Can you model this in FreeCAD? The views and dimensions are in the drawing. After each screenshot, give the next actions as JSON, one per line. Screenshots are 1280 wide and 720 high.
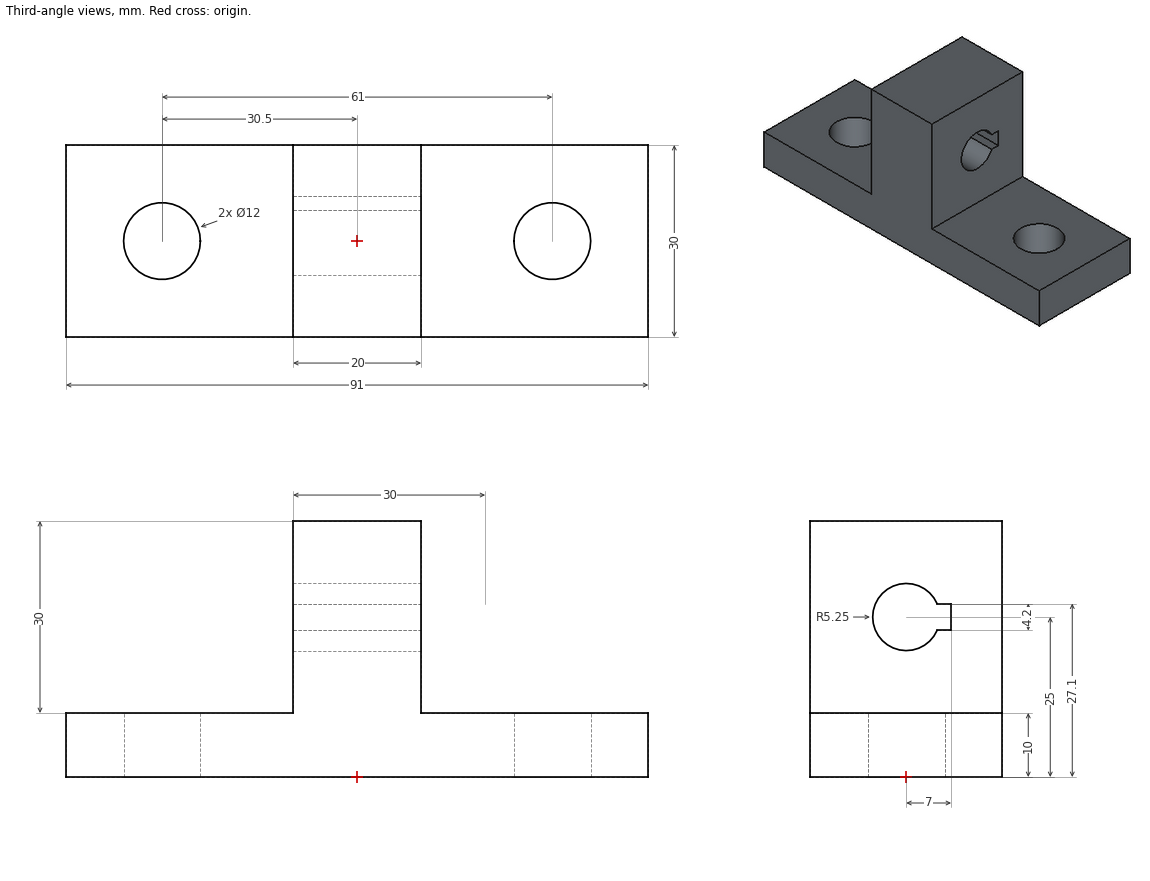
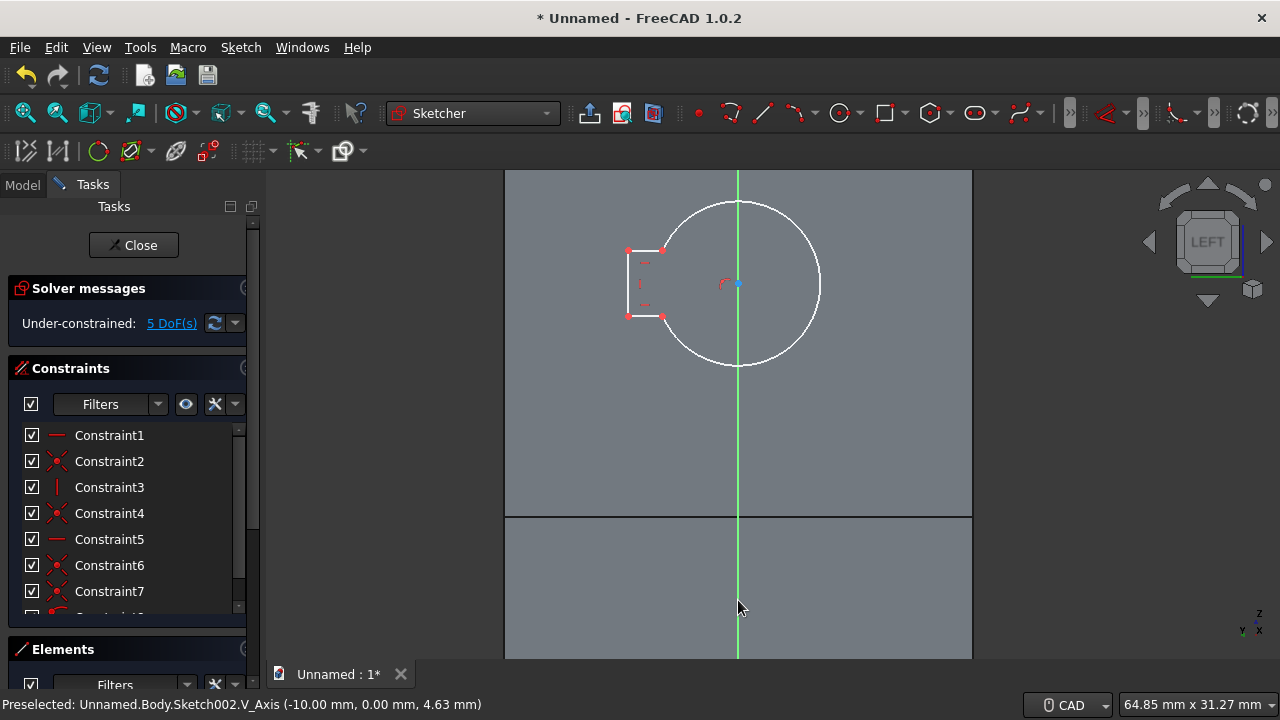
{"action": "left_click", "coordinate": [1106, 114]}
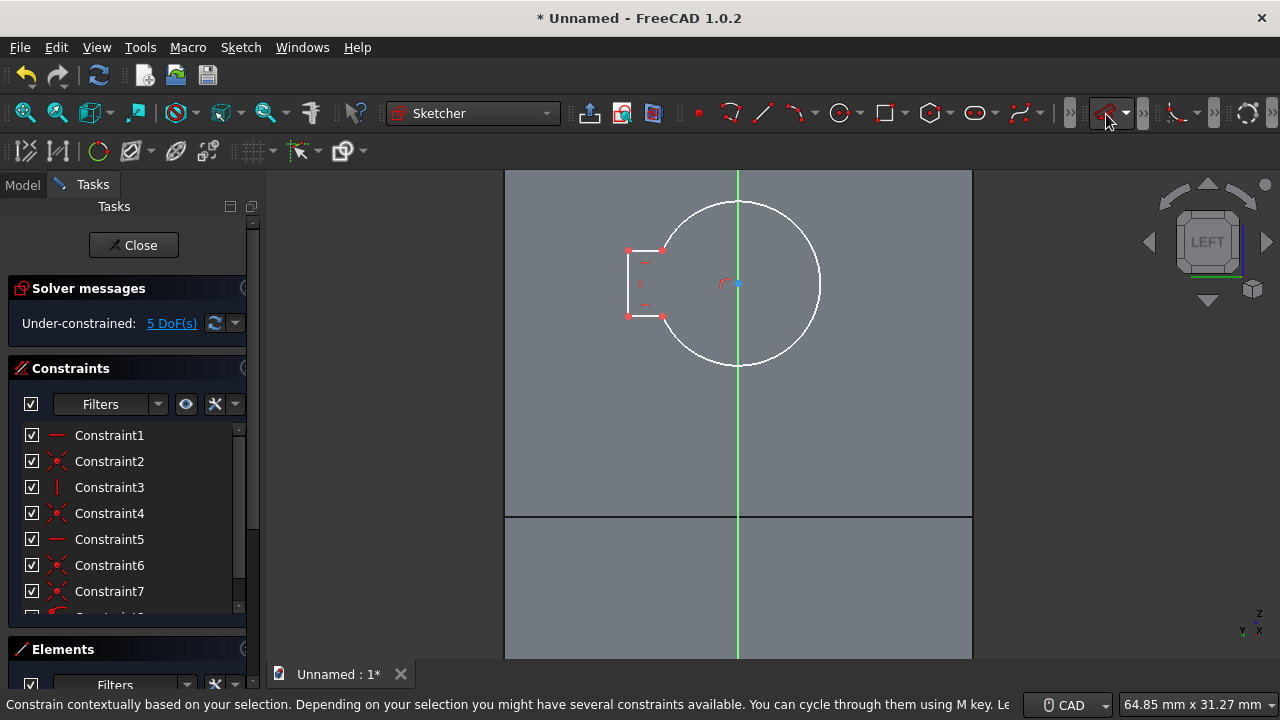
{"action": "left_click", "coordinate": [776, 356]}
{"action": "left_click", "coordinate": [791, 384]}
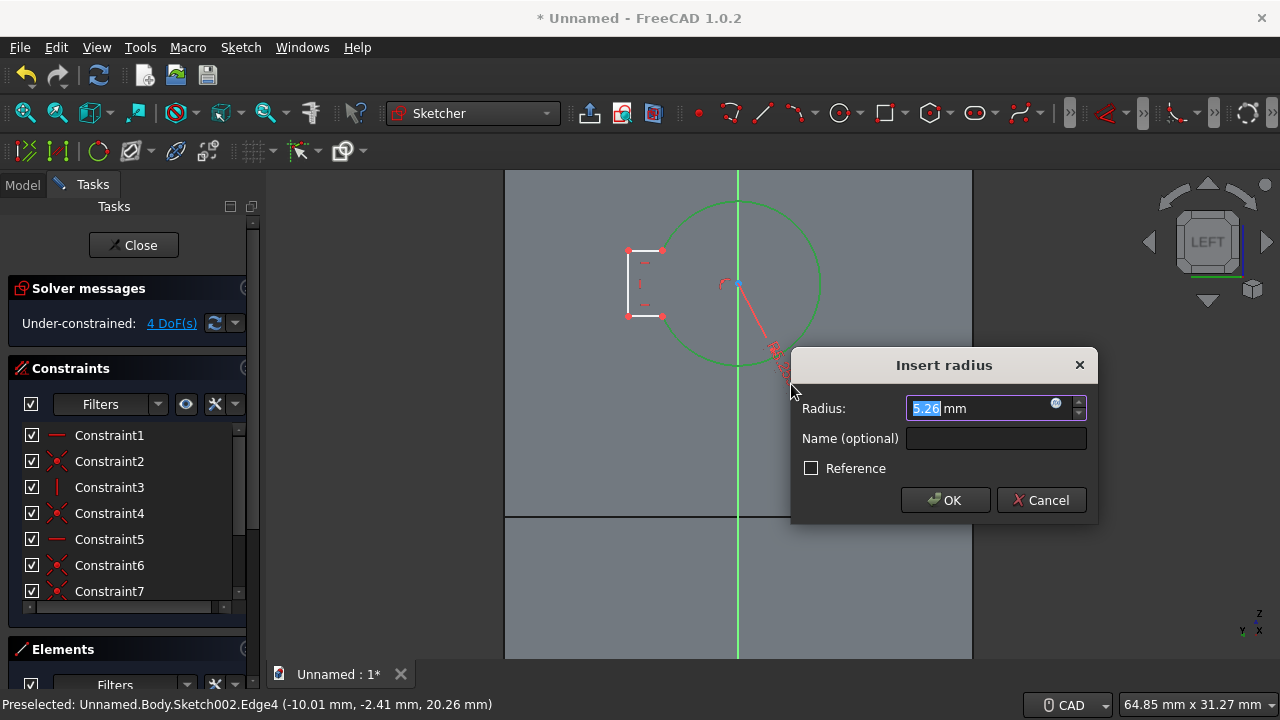
{"action": "type", "text": "5.25"}
{"action": "key", "text": "Return"}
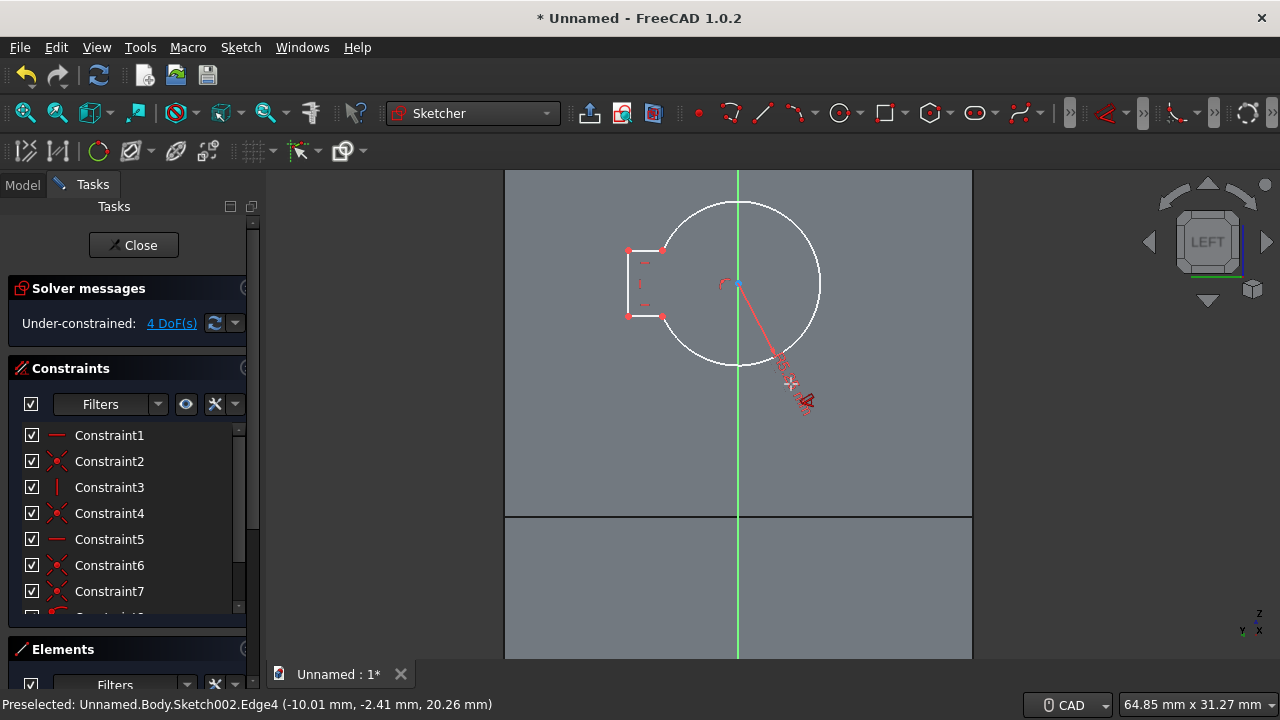
{"action": "left_click", "coordinate": [628, 251]}
{"action": "left_click", "coordinate": [658, 217]}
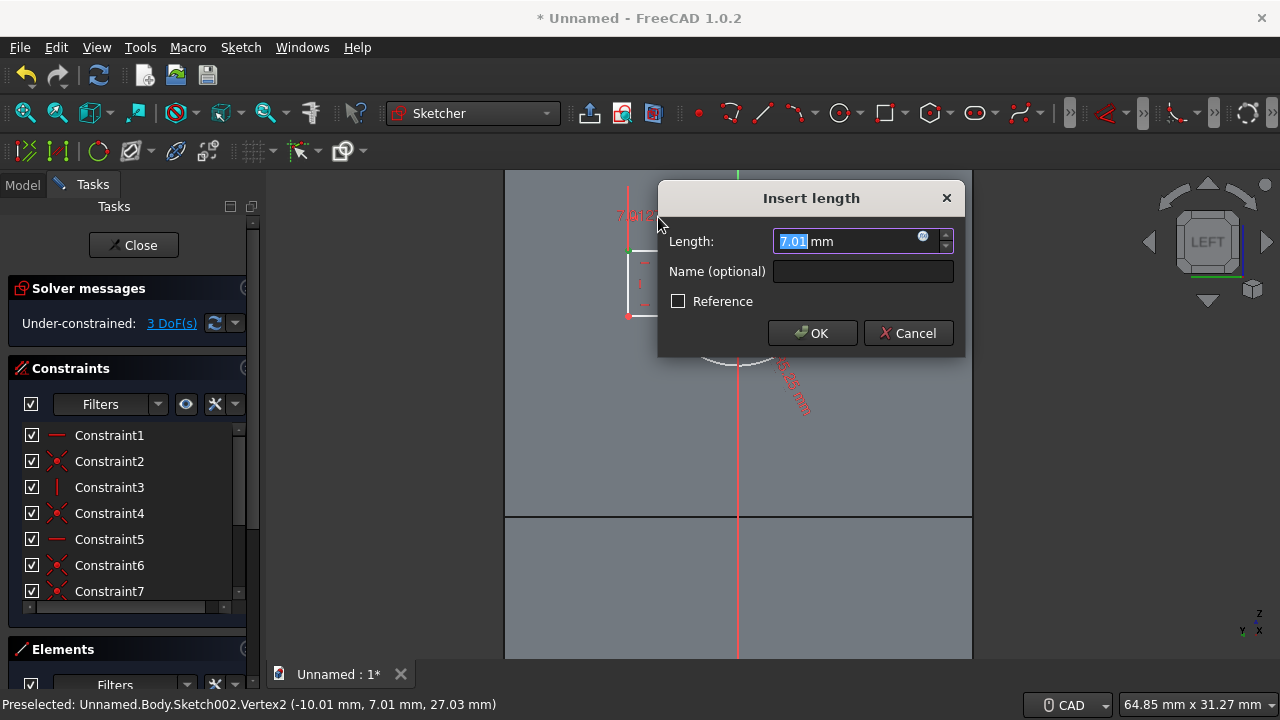
{"action": "type", "text": "7"}
{"action": "key", "text": "Return"}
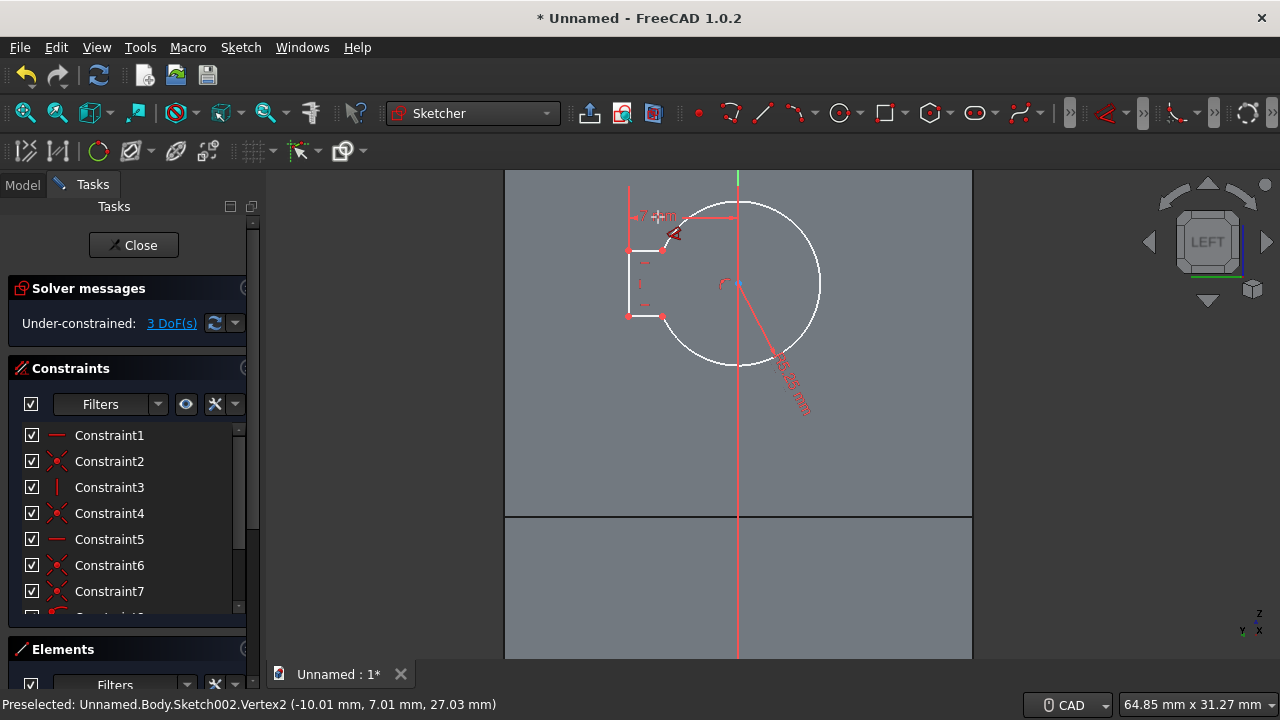
{"action": "left_click", "coordinate": [629, 270]}
{"action": "left_click", "coordinate": [595, 284]}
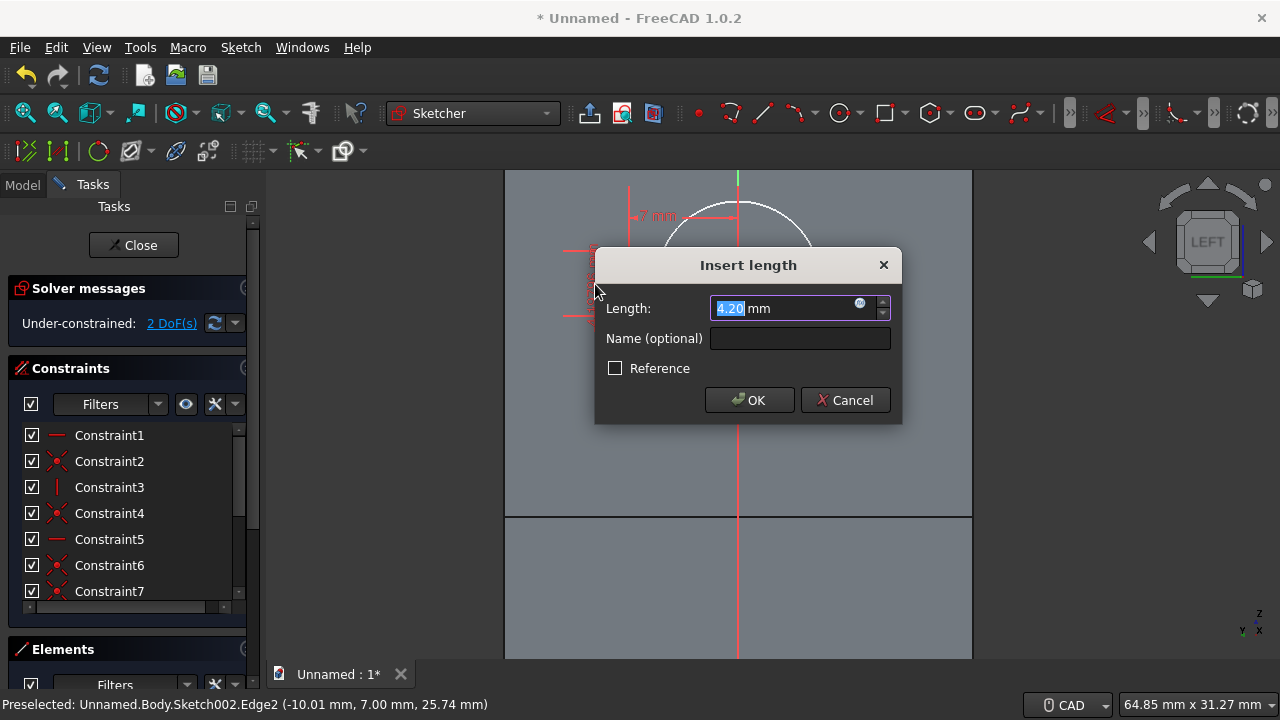
{"action": "type", "text": "4.2"}
{"action": "key", "text": "Return"}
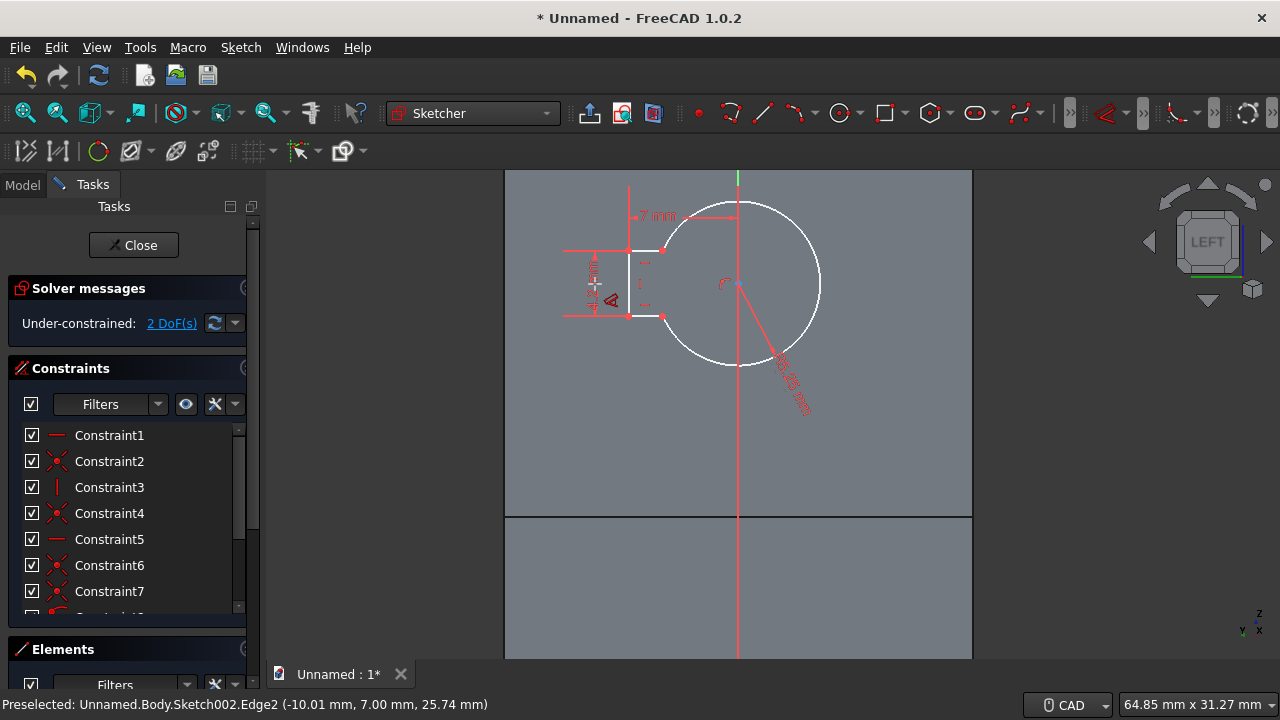
{"action": "left_click", "coordinate": [738, 284]}
{"action": "left_click", "coordinate": [772, 457]}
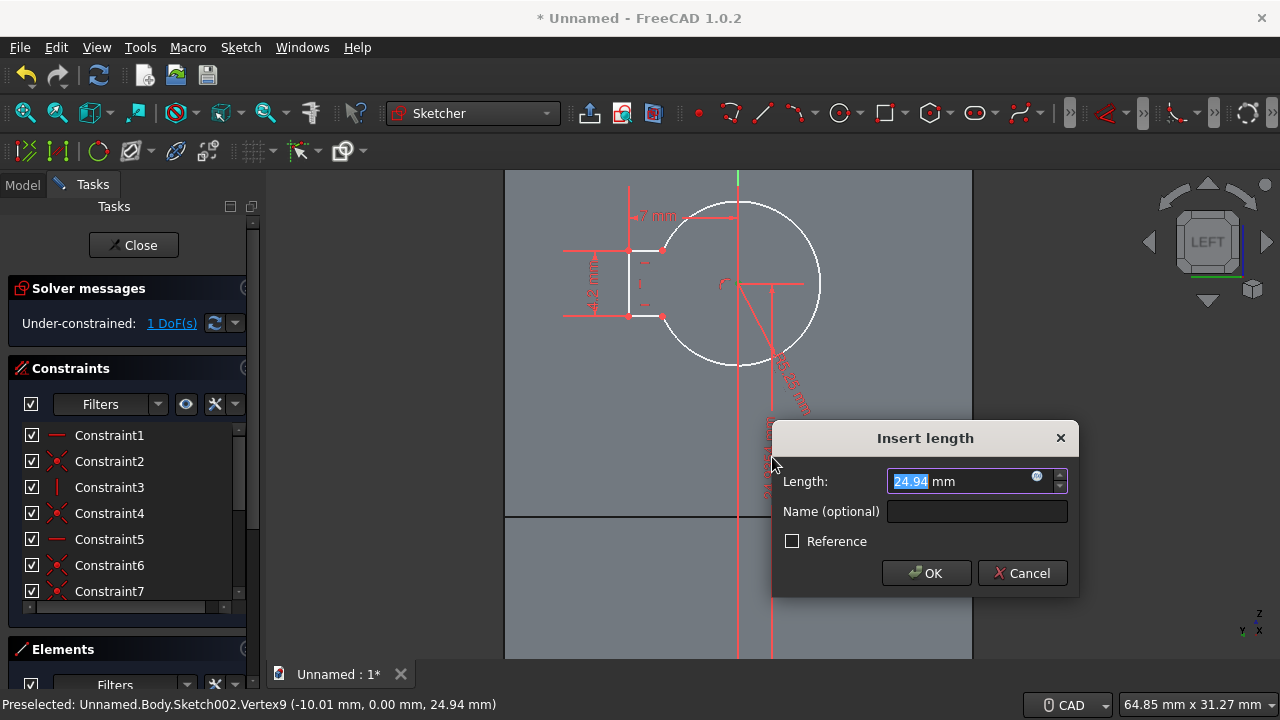
{"action": "type", "text": "25"}
{"action": "key", "text": "Return"}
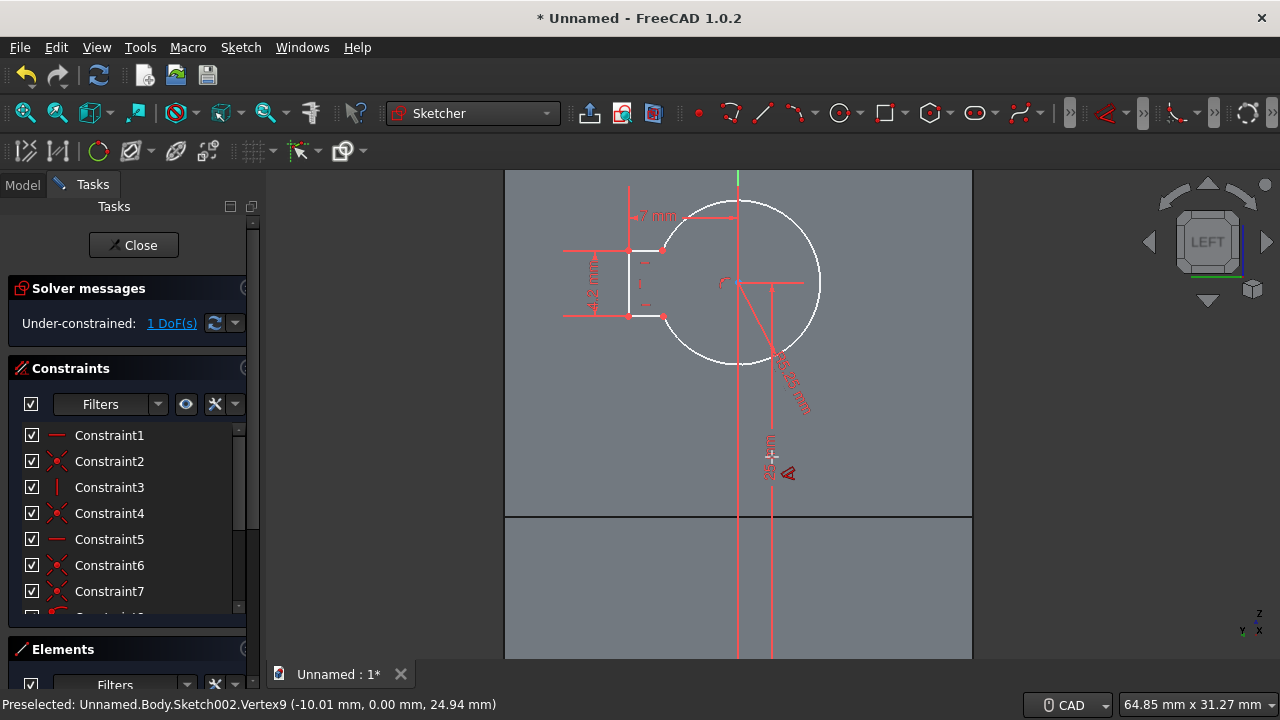
{"action": "left_click", "coordinate": [662, 251]}
{"action": "left_click", "coordinate": [628, 441]}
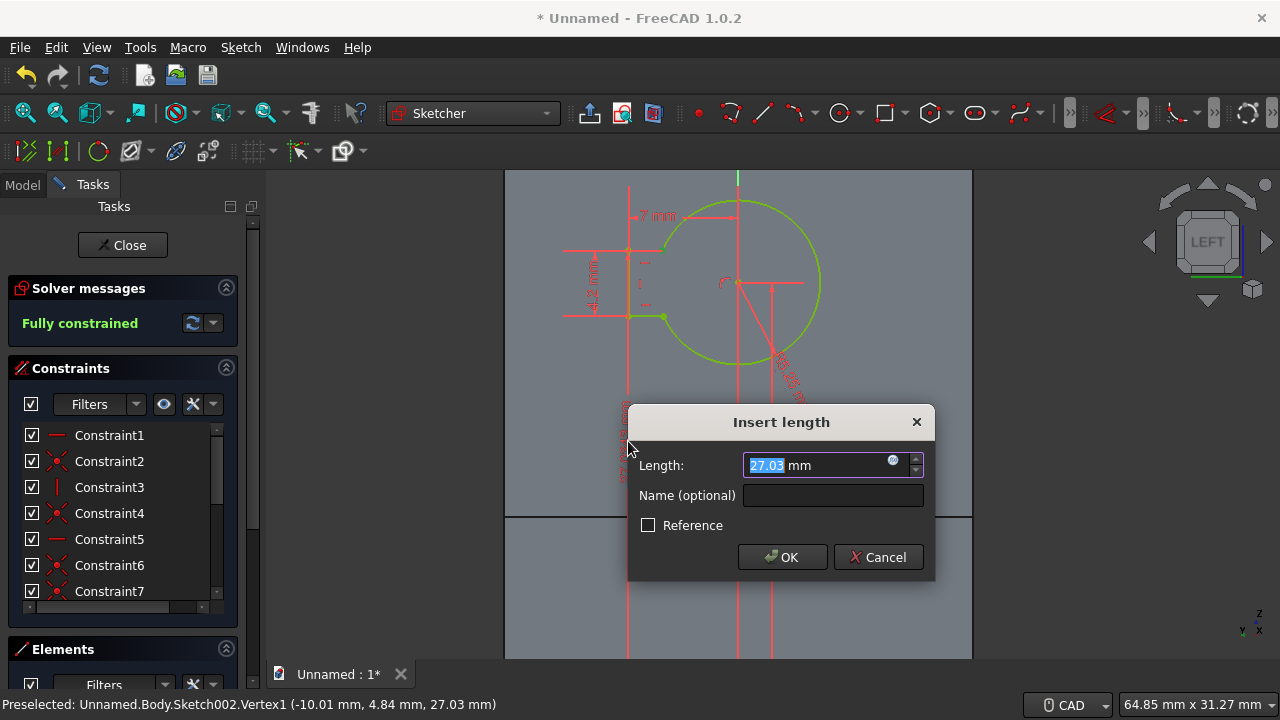
{"action": "type", "text": "27.1"}
{"action": "key", "text": "Return"}
{"action": "key", "text": "Escape"}